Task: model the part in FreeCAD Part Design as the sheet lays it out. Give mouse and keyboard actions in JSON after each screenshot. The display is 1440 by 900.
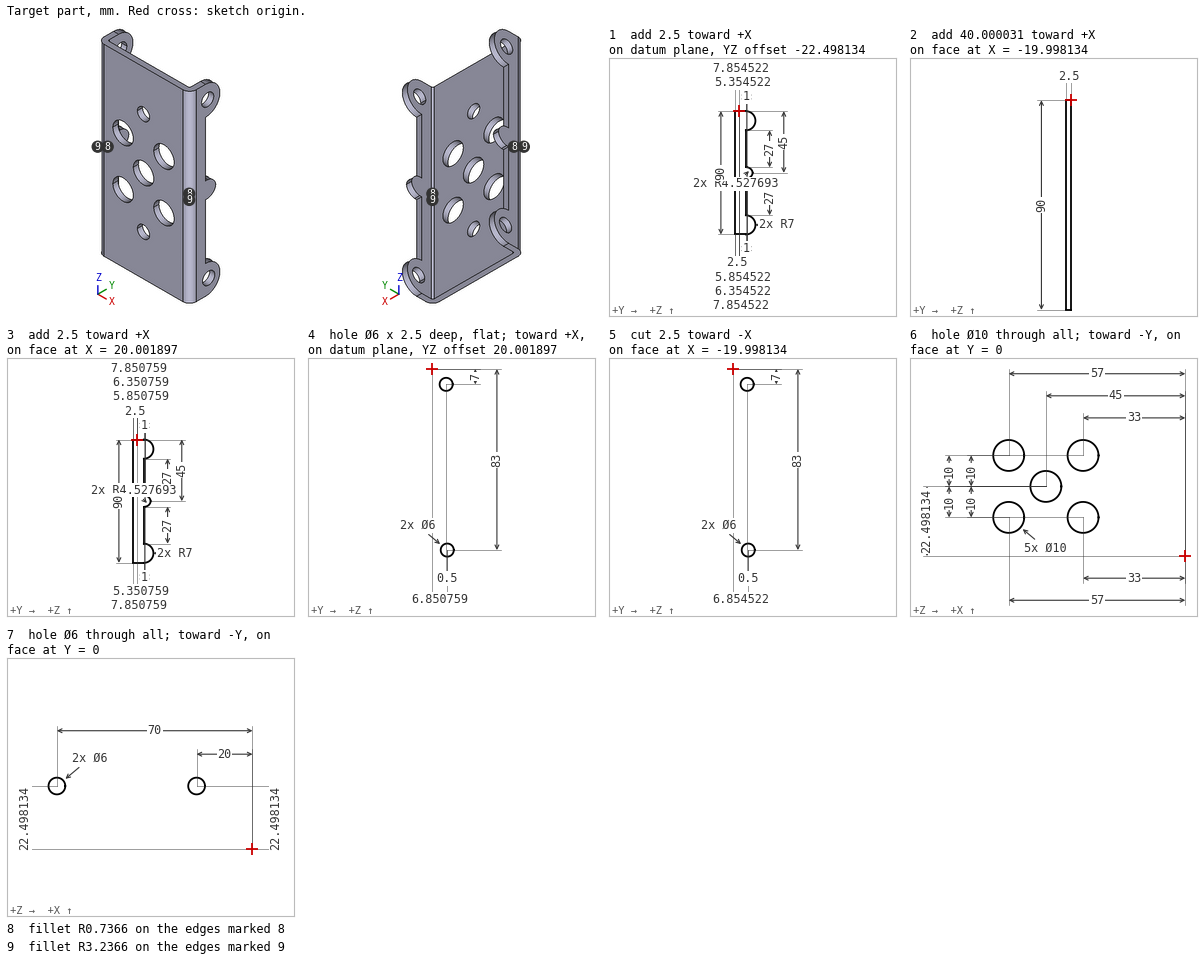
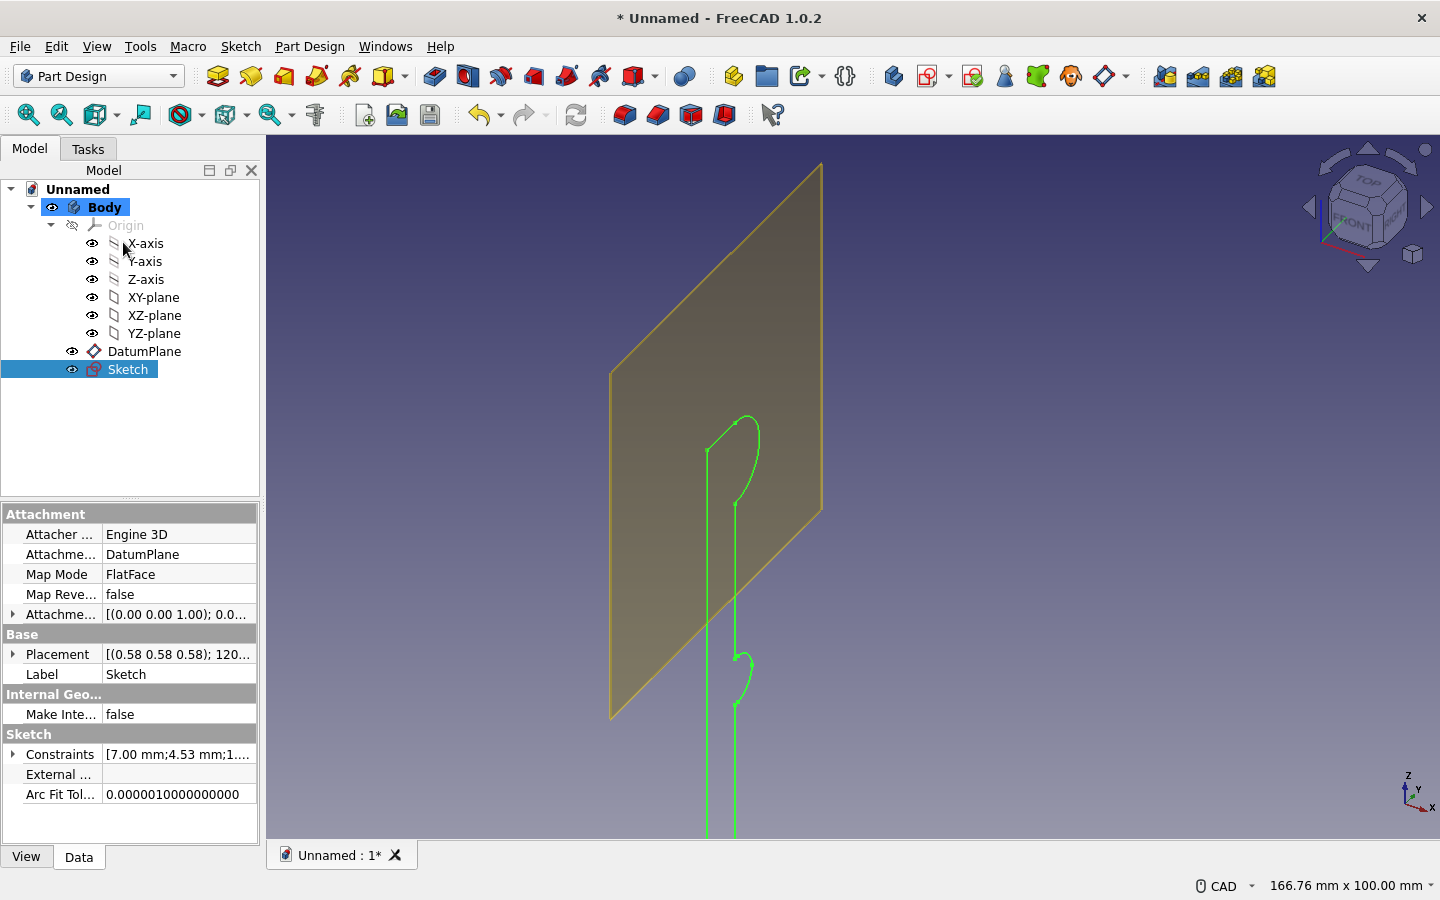
{"action": "left_click", "coordinate": [218, 76]}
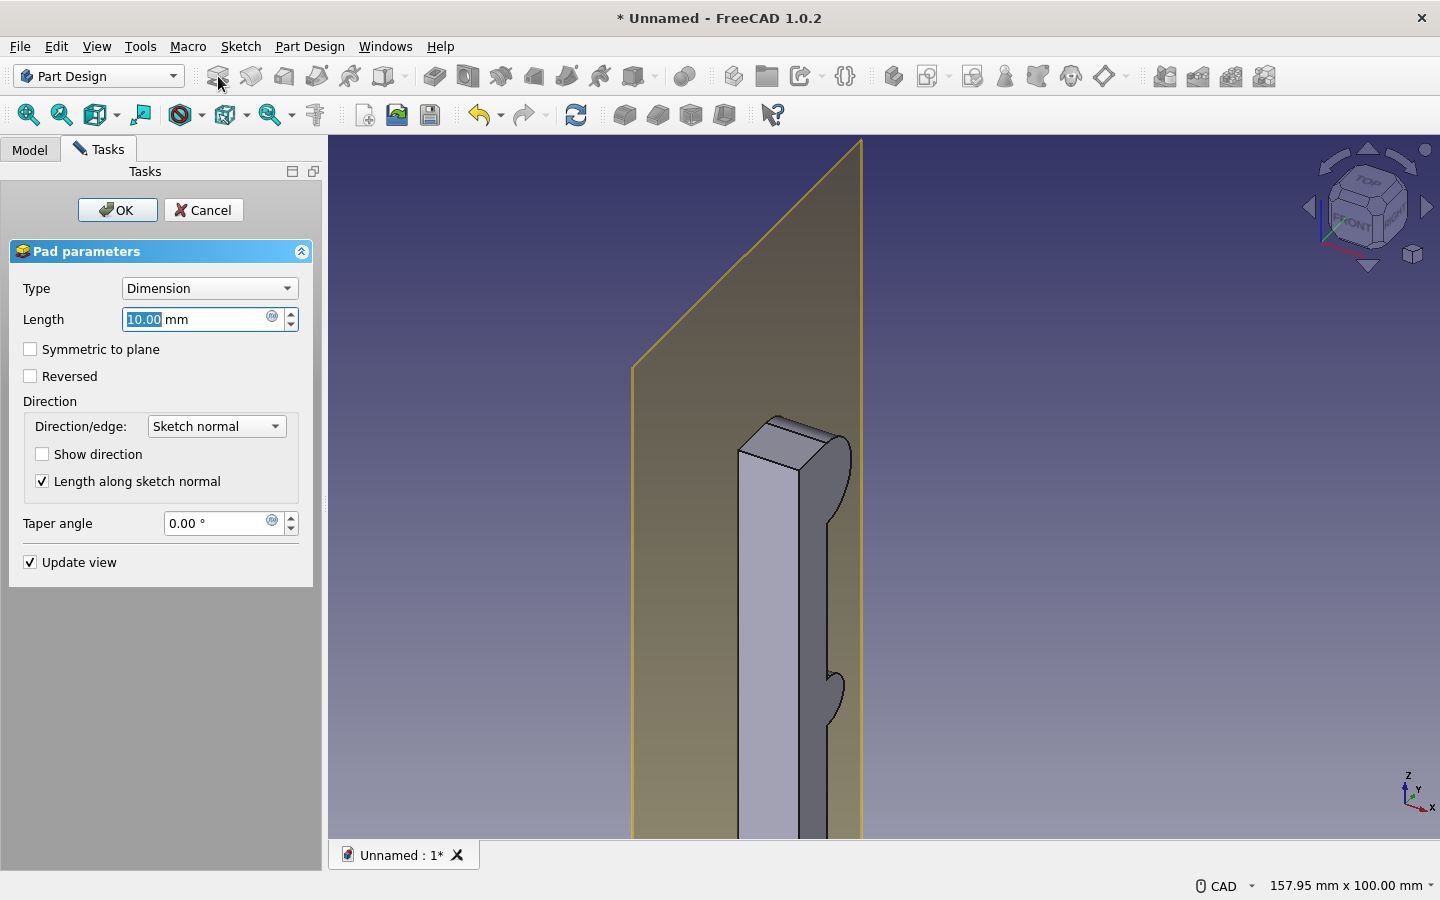
{"action": "type", "text": "2.5"}
{"action": "key", "text": "Tab"}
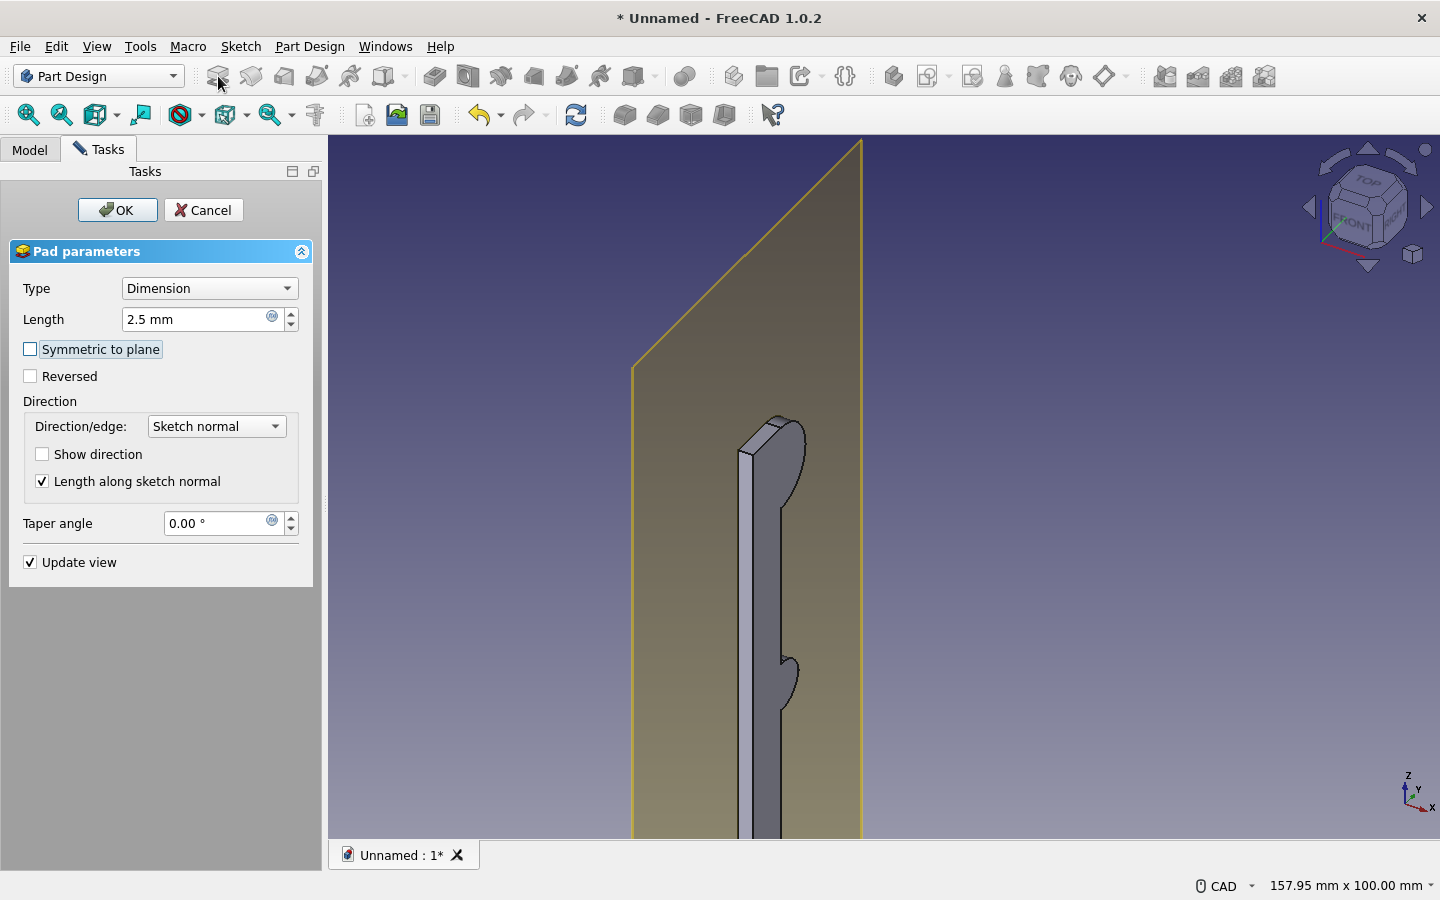
{"action": "left_click", "coordinate": [118, 210]}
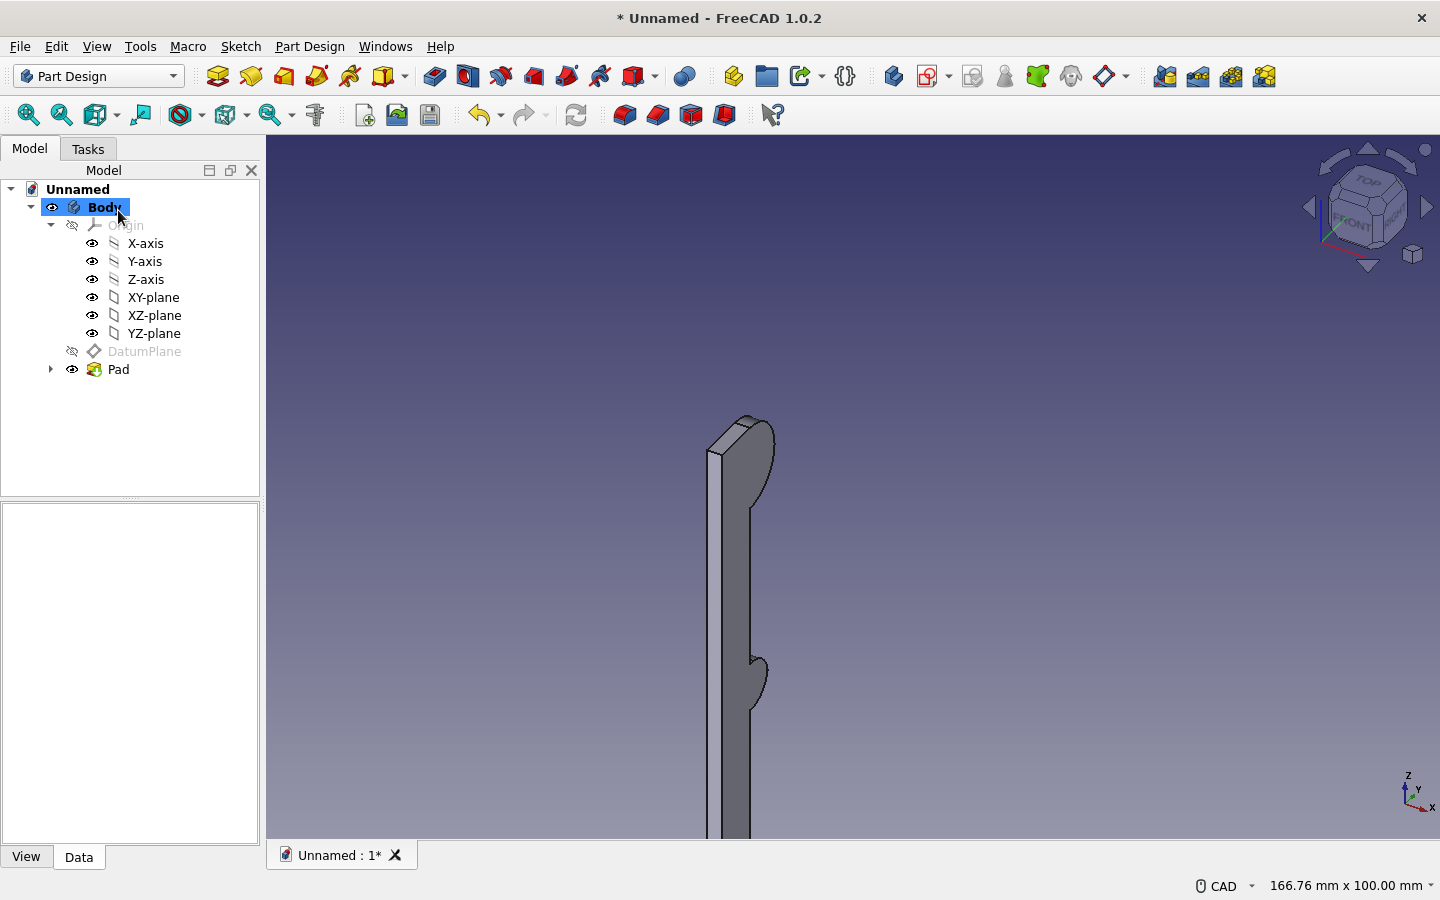
{"action": "key", "text": "v f"}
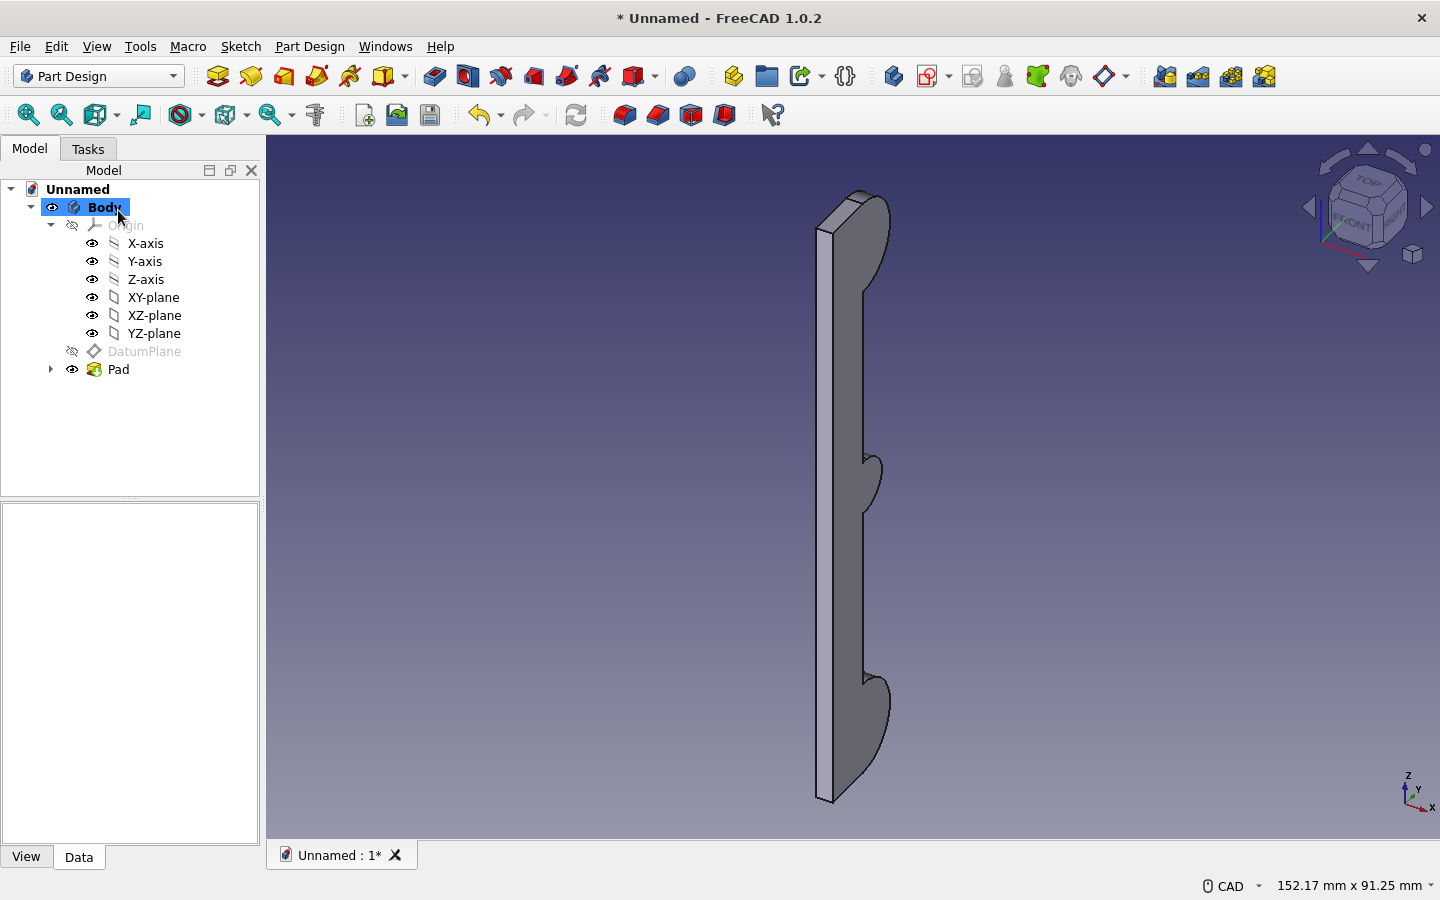
{"action": "left_click", "coordinate": [861, 733]}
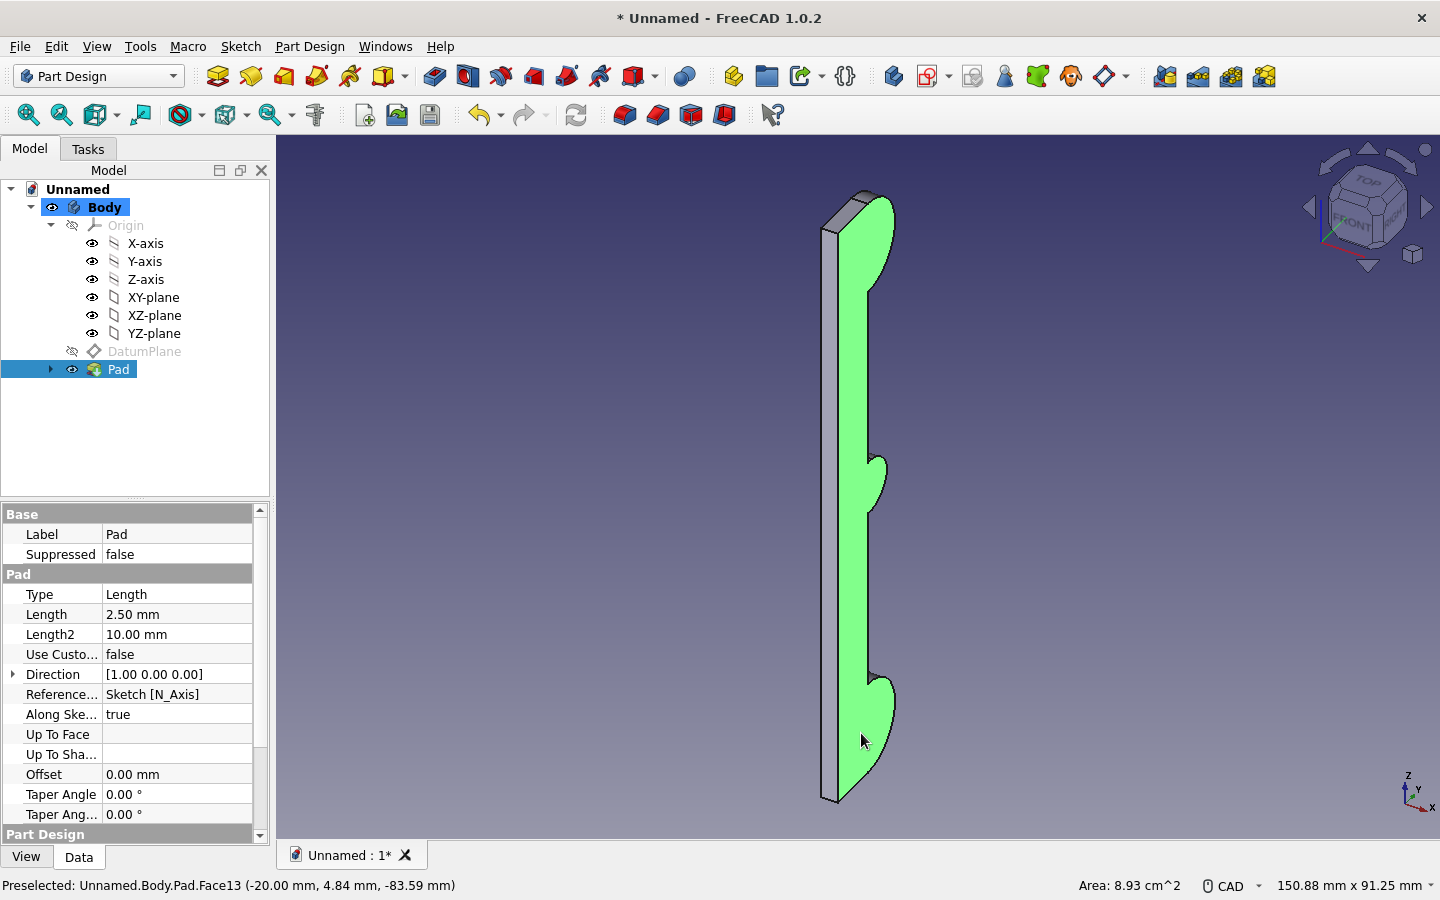
{"action": "left_click", "coordinate": [926, 76]}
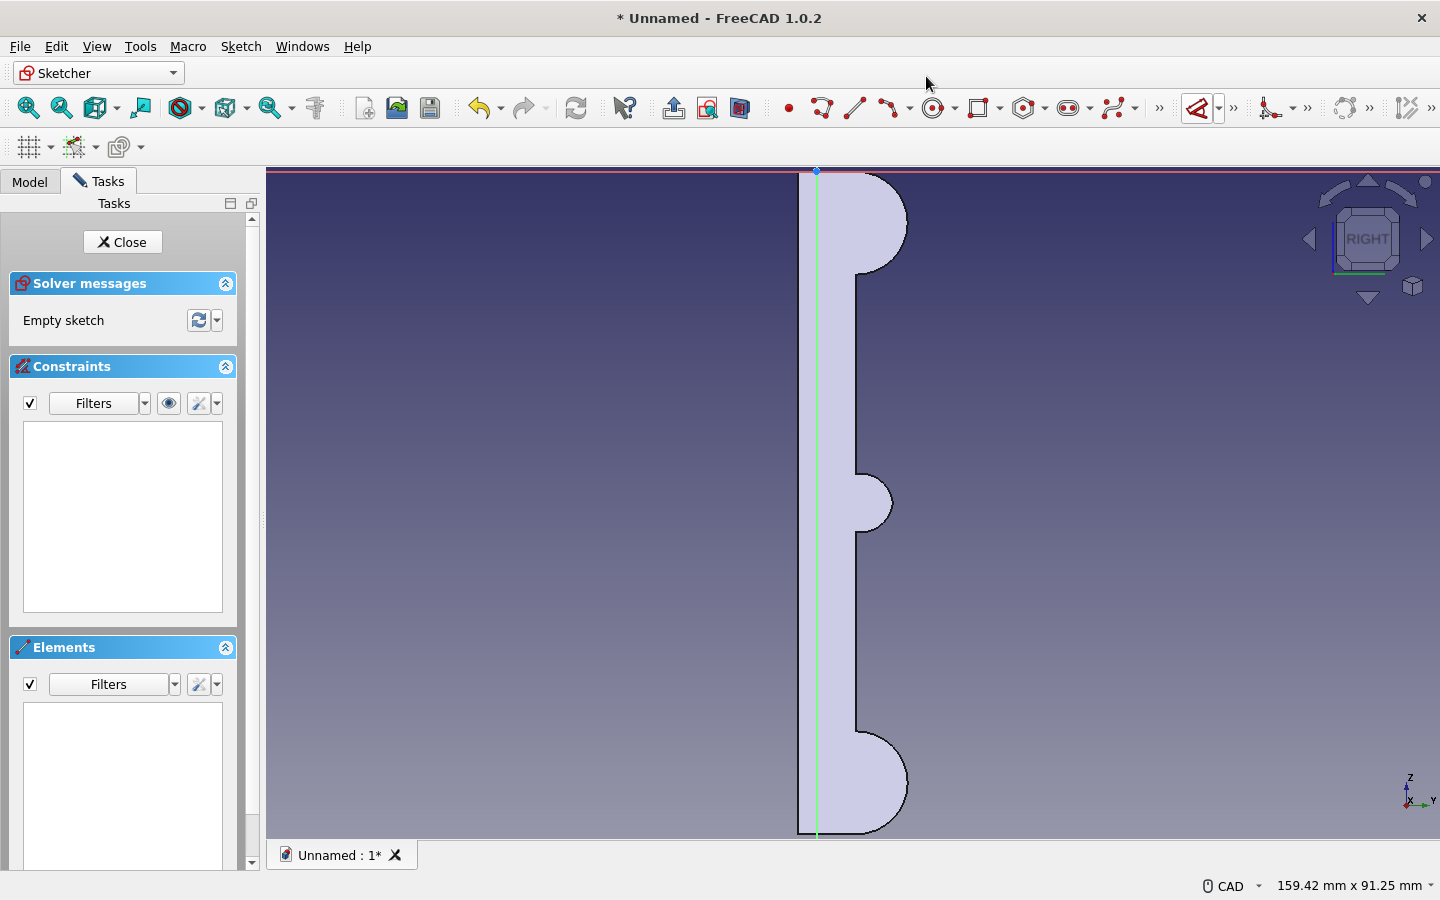
{"action": "scroll", "coordinate": [738, 503], "scroll_direction": "down", "scroll_amount": 2}